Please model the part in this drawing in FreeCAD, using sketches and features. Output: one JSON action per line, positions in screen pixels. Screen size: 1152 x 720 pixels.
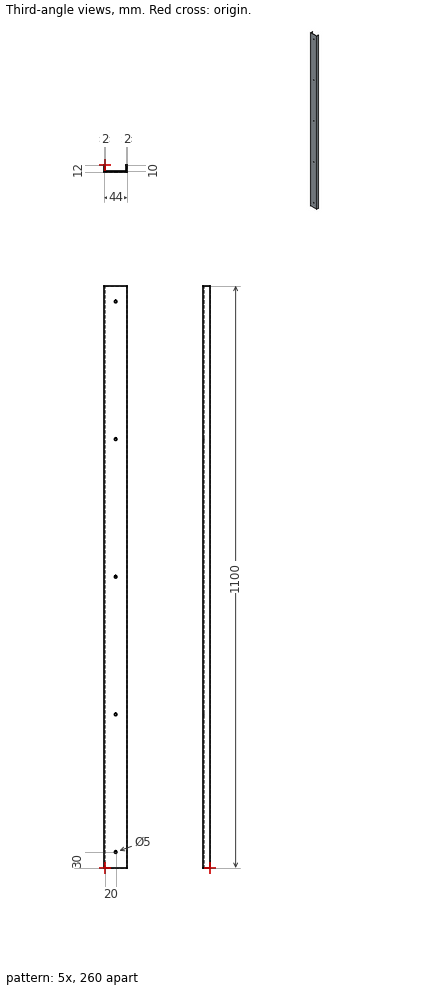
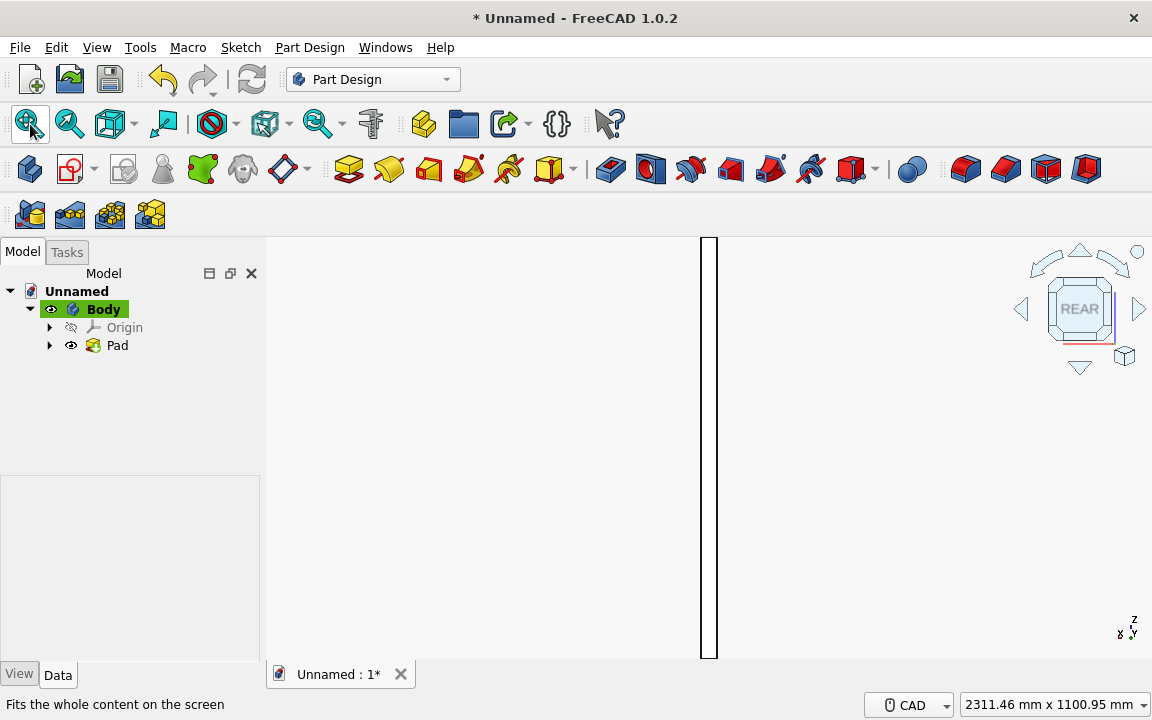
{"action": "left_click", "coordinate": [30, 124]}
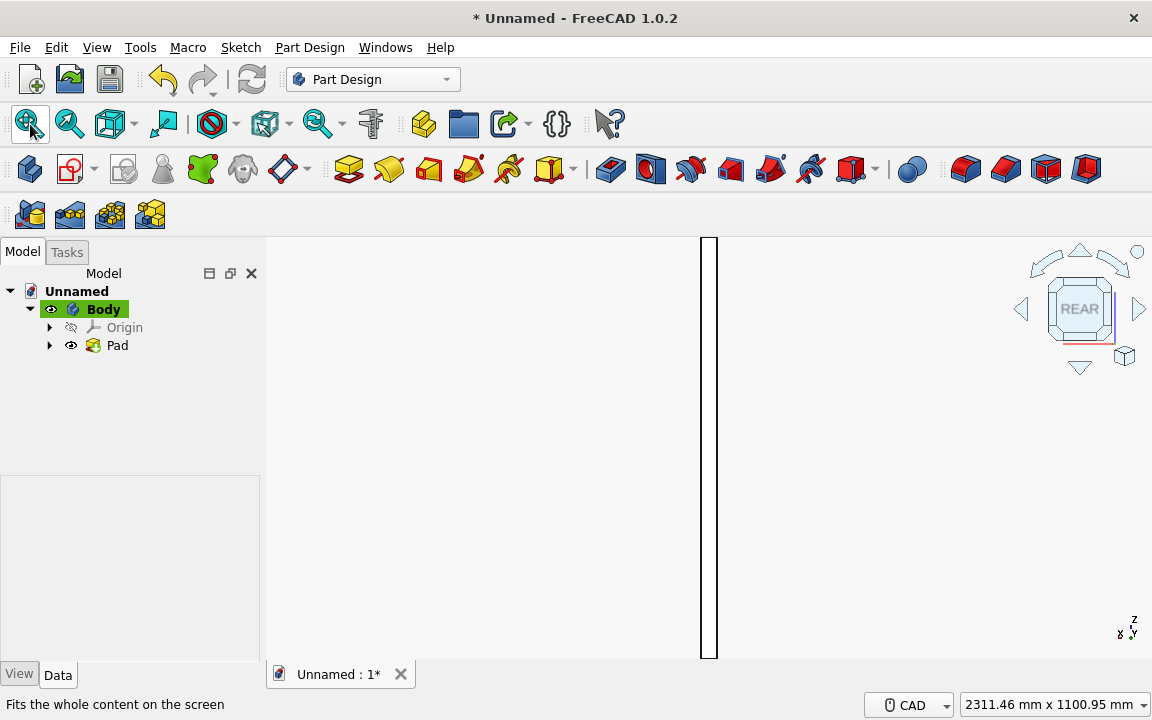
{"action": "key", "text": "2"}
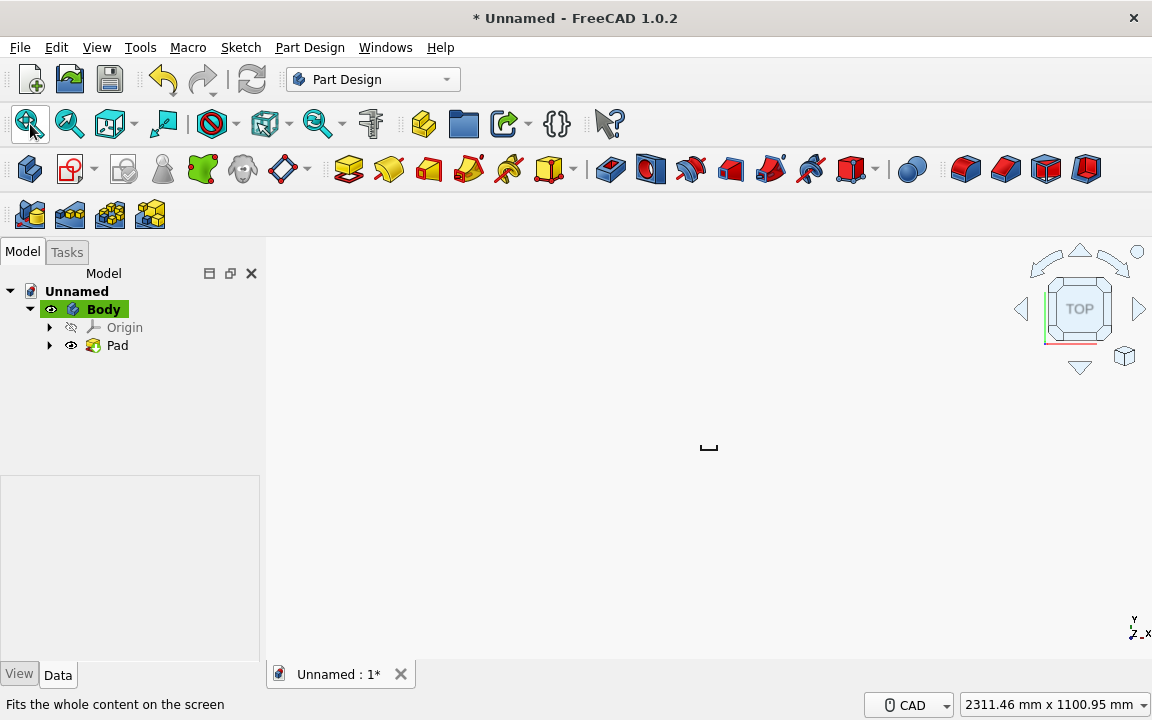
{"action": "left_click", "coordinate": [30, 124]}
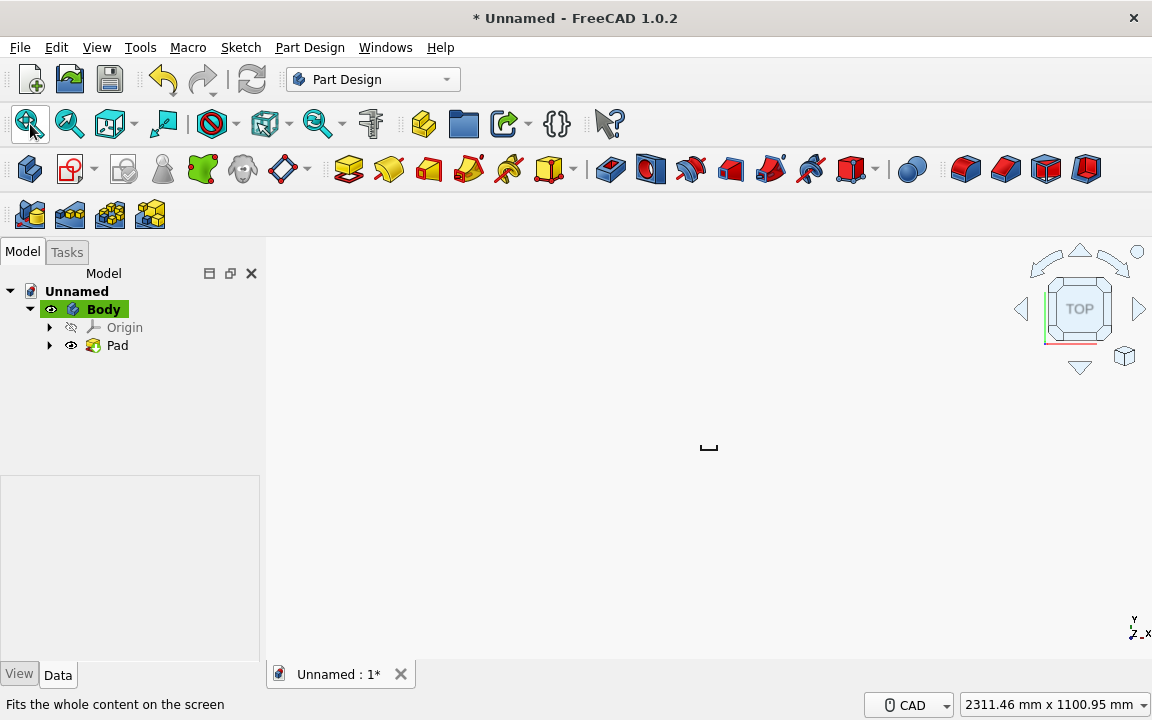
{"action": "key", "text": "3"}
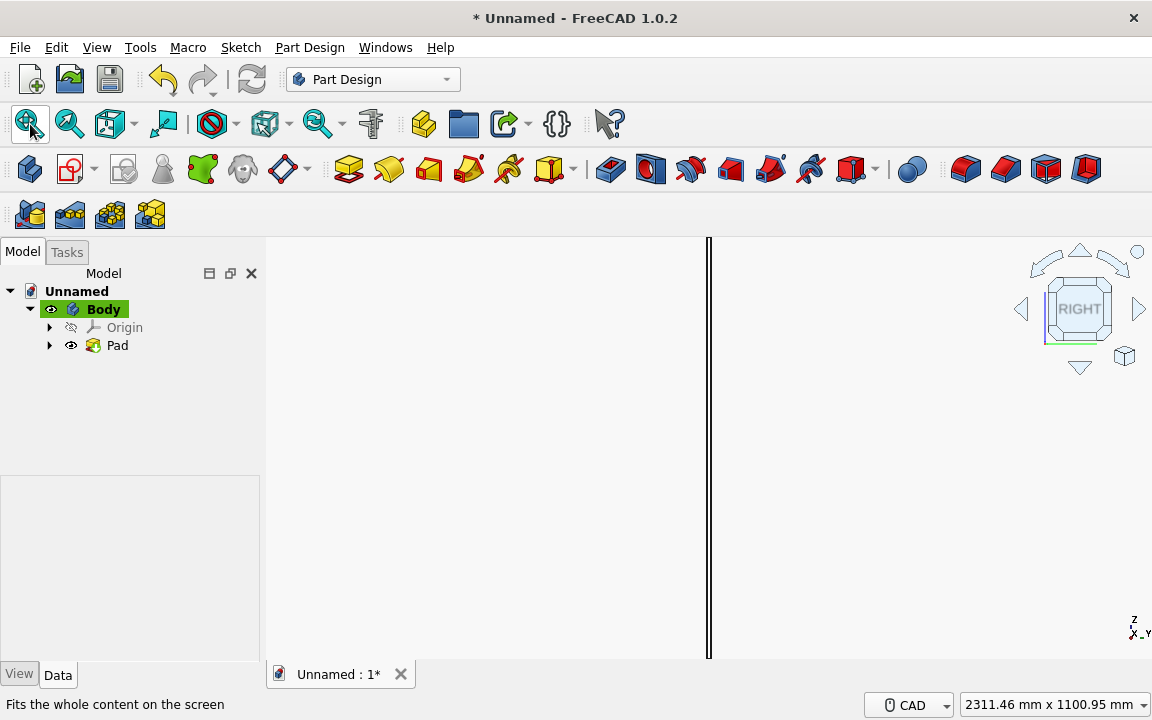
{"action": "left_click", "coordinate": [30, 124]}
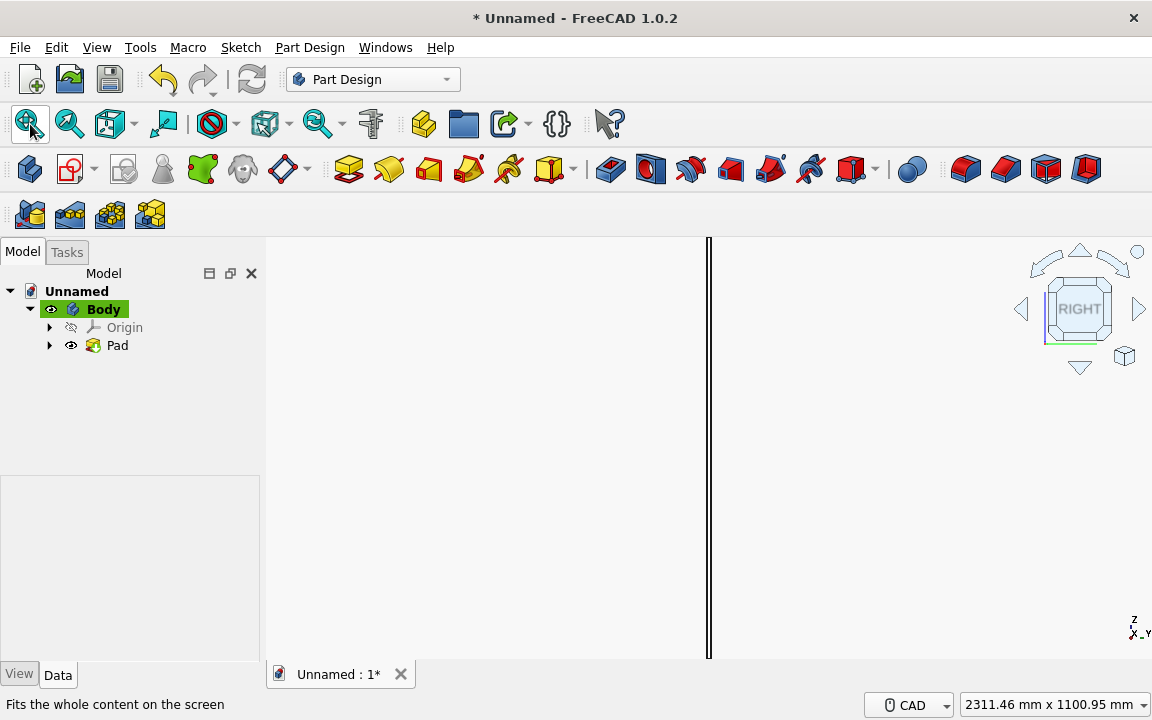
{"action": "left_click", "coordinate": [50, 327]}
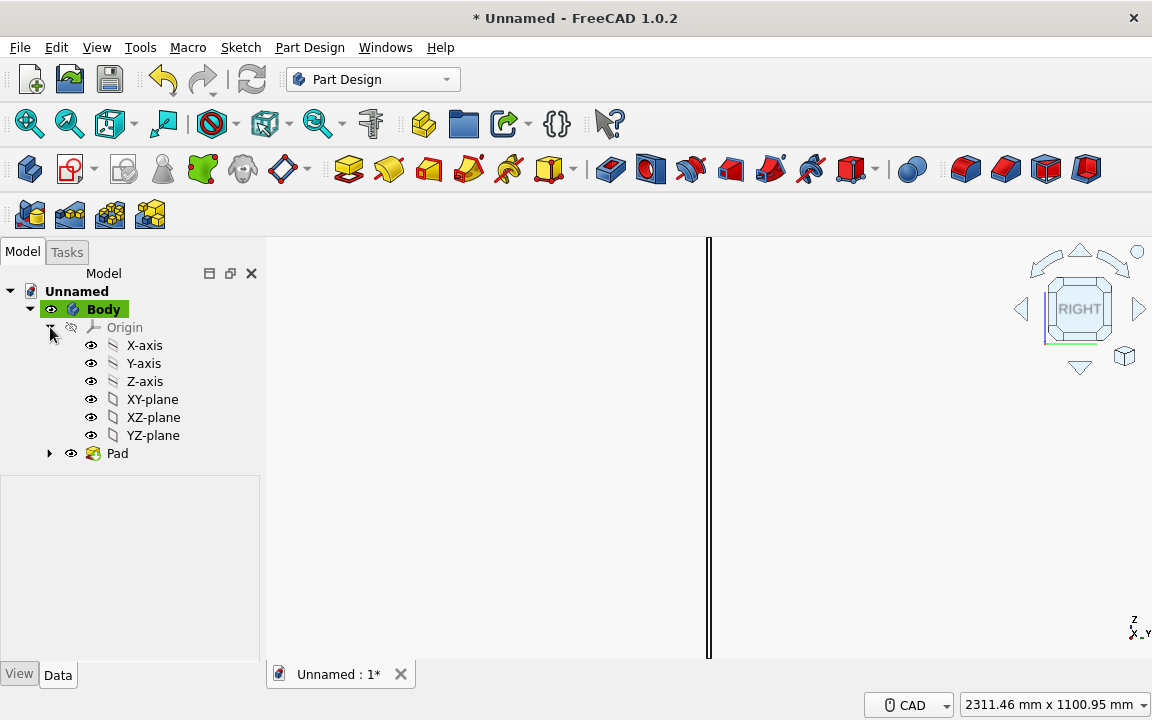
{"action": "left_click", "coordinate": [136, 417]}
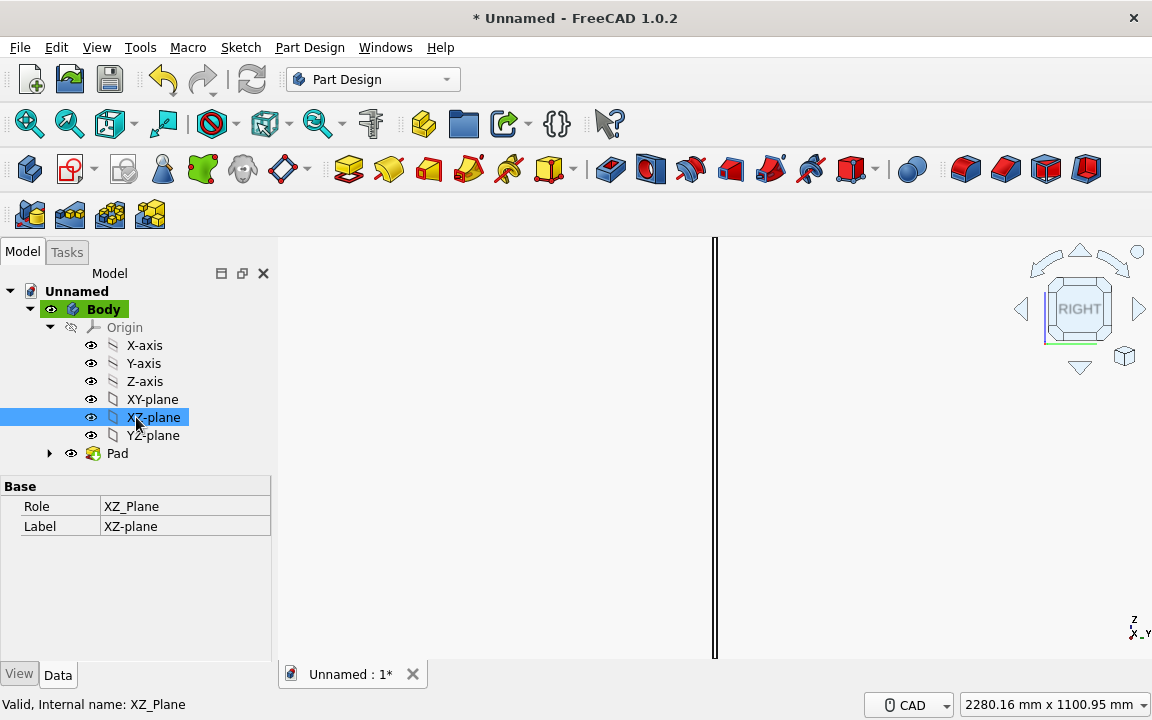
{"action": "left_click", "coordinate": [284, 170]}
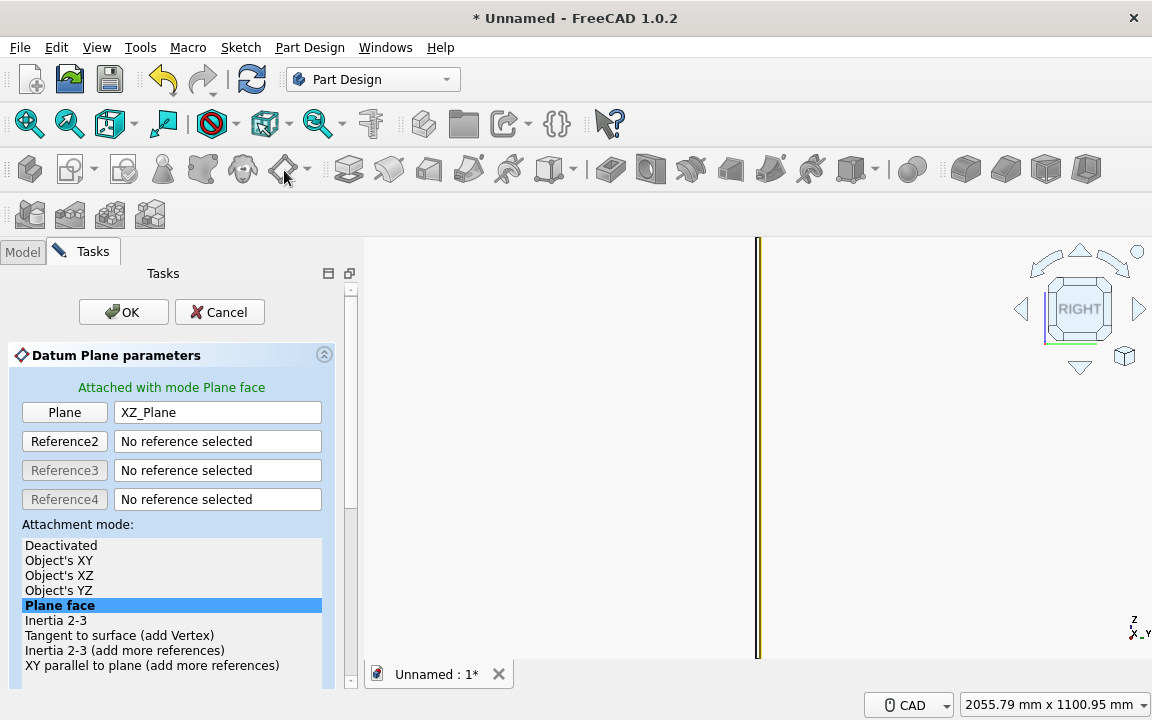
{"action": "scroll", "coordinate": [351, 486], "scroll_direction": "down", "scroll_amount": 4}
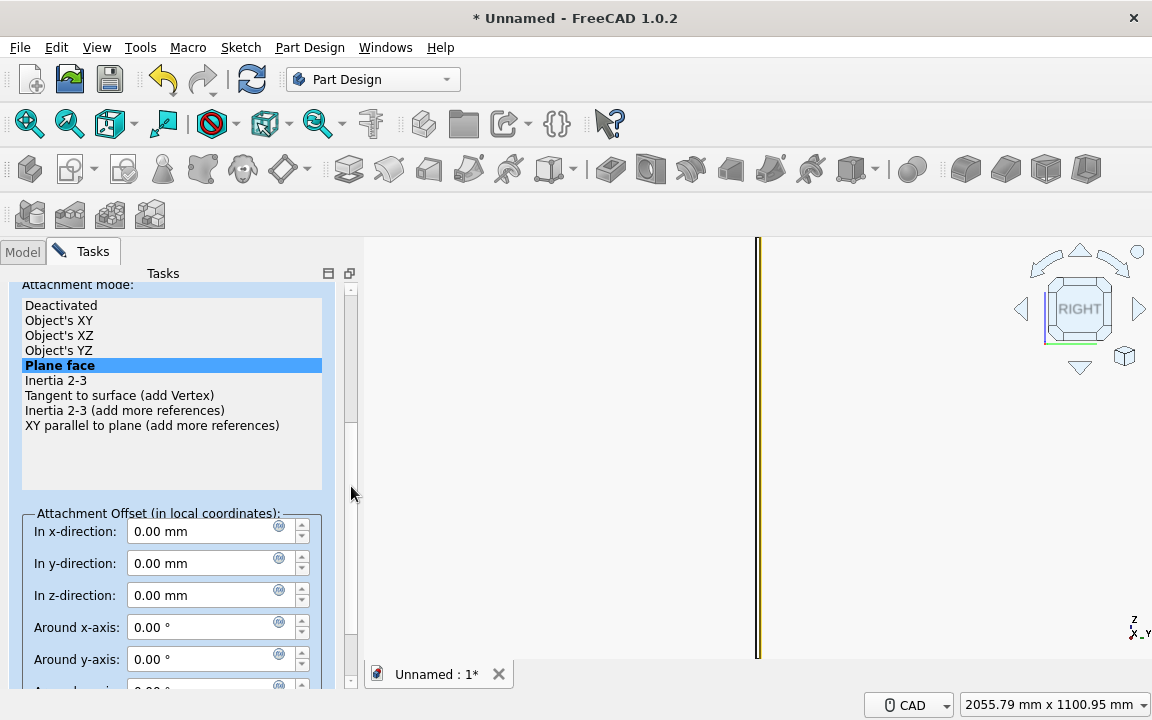
{"action": "triple_click", "coordinate": [210, 595]}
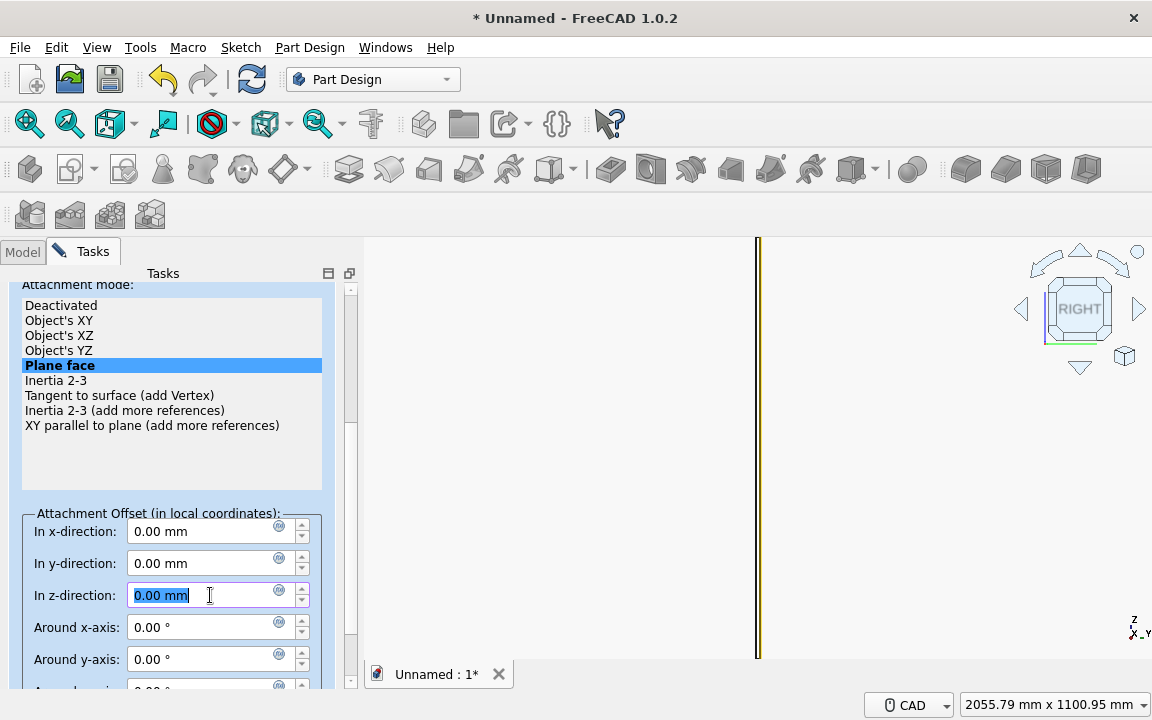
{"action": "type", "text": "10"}
{"action": "key", "text": "Tab"}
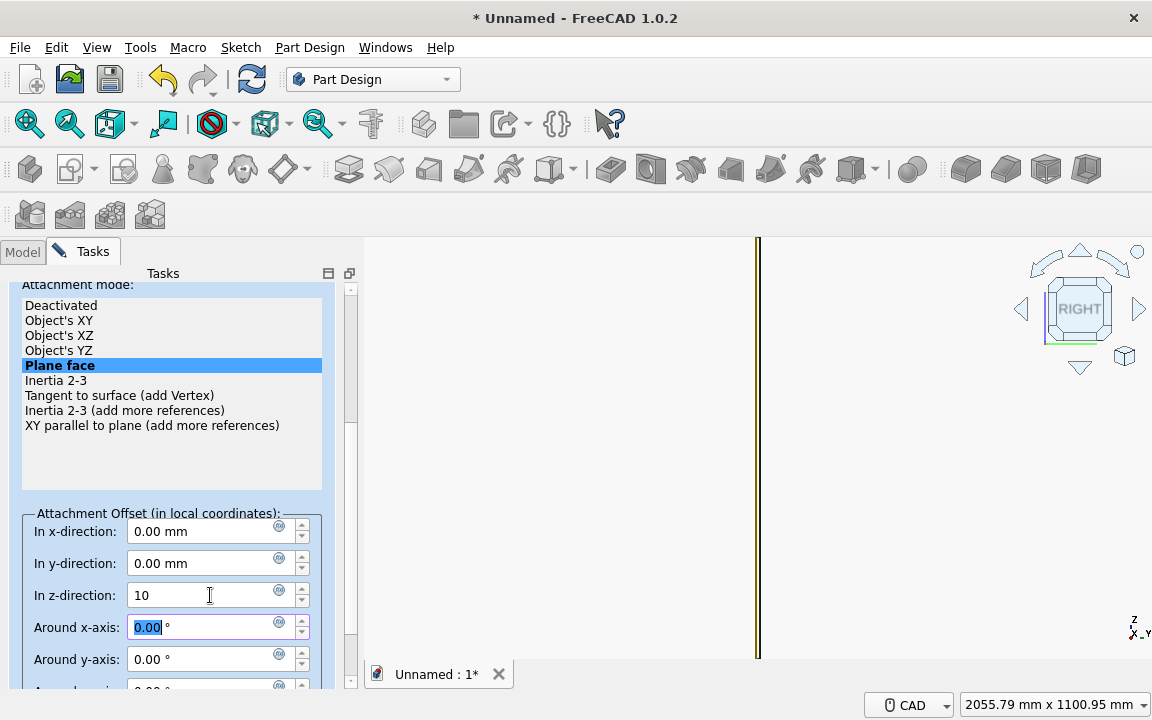
{"action": "scroll", "coordinate": [351, 486], "scroll_direction": "up", "scroll_amount": 5}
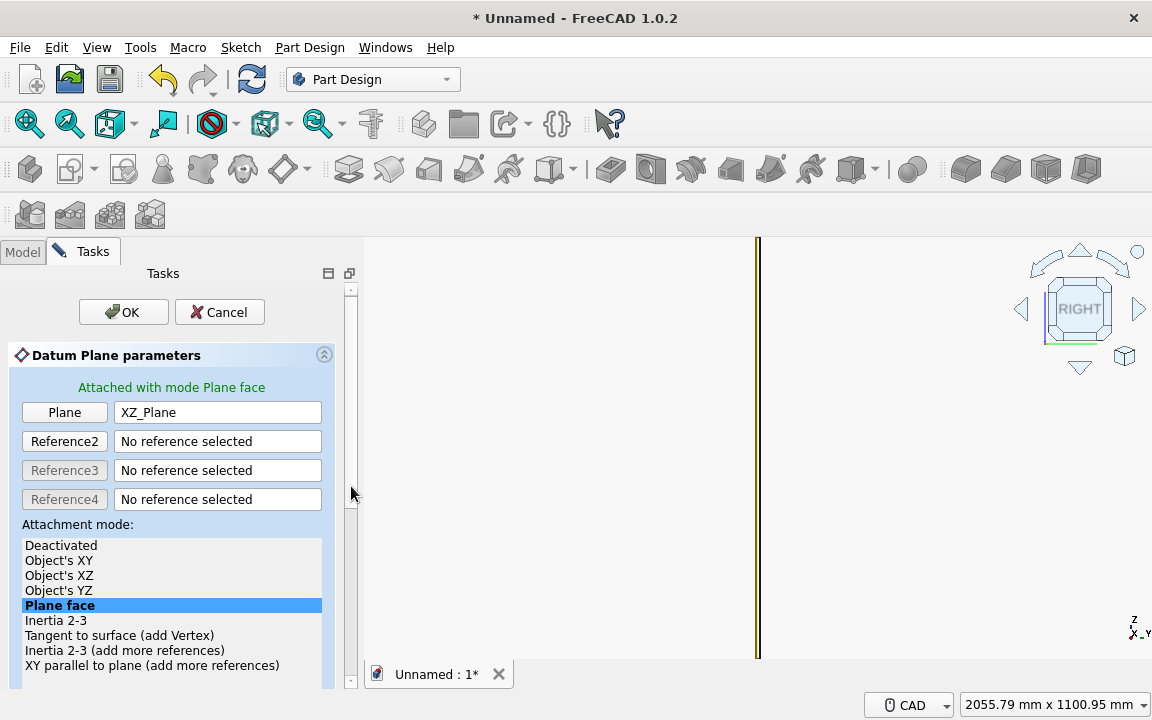
{"action": "left_click", "coordinate": [124, 312]}